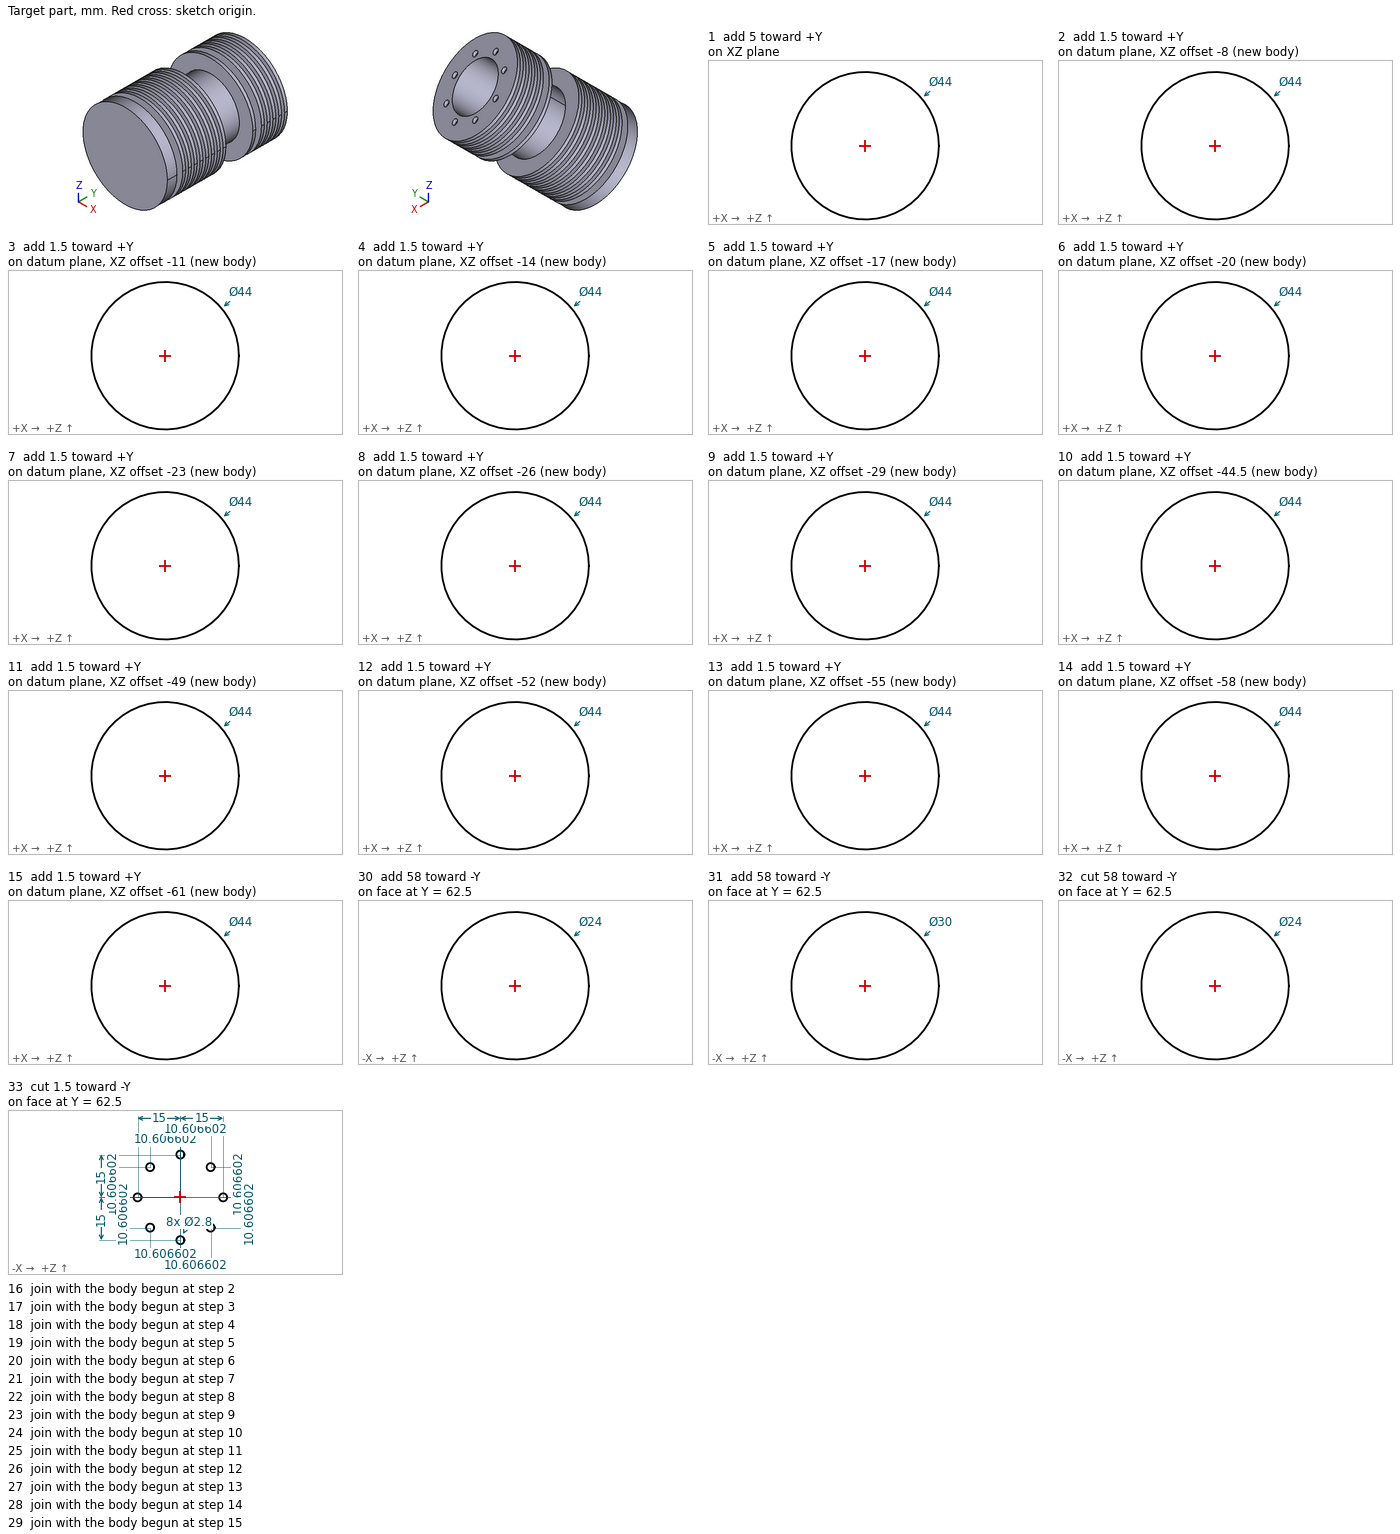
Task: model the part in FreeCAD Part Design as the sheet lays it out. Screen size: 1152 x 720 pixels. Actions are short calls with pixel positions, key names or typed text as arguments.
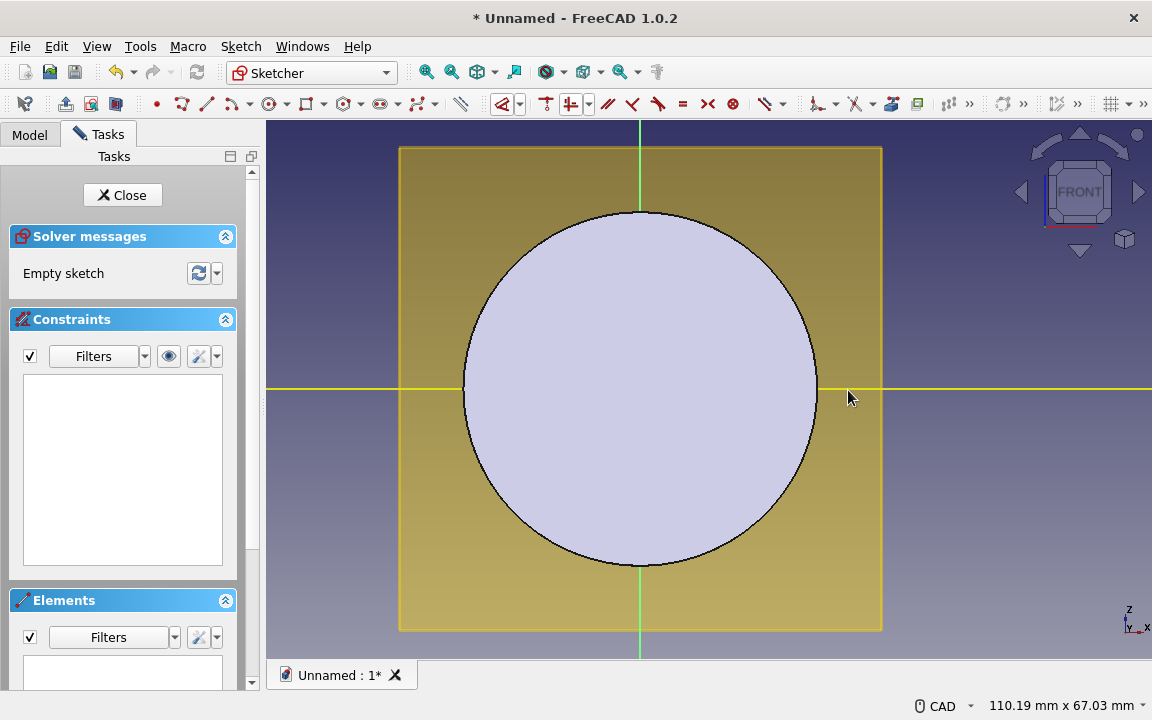
key(g)
key(c)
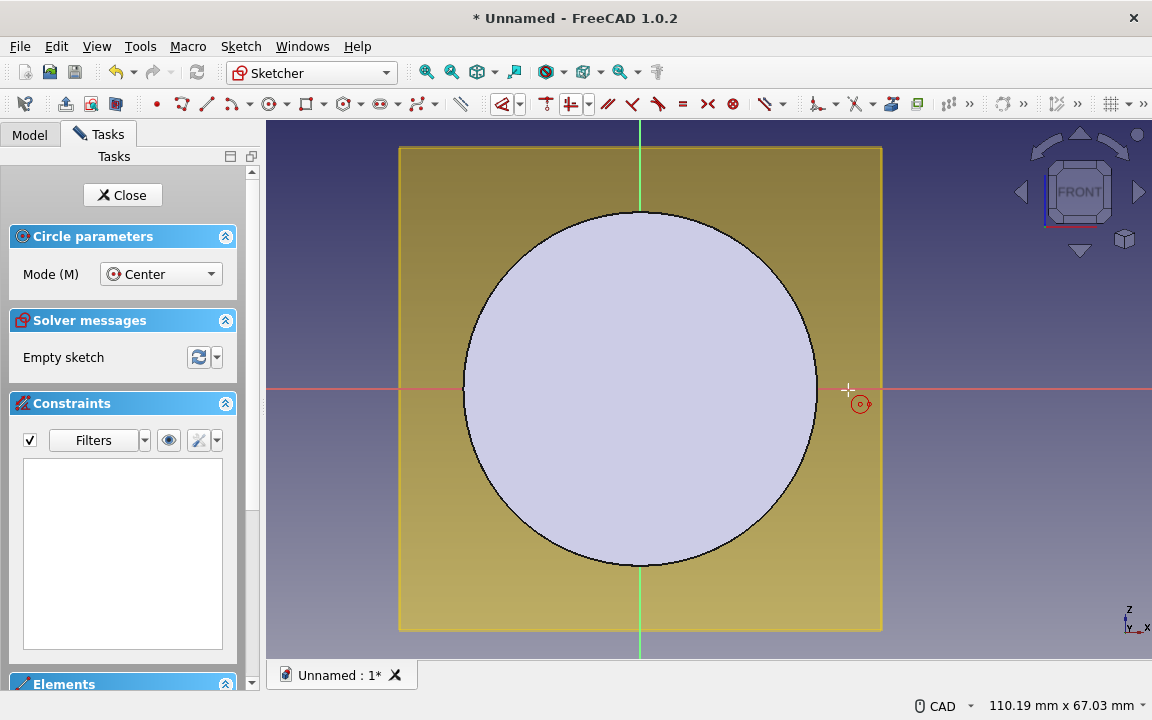
click(640, 389)
click(765, 264)
key(Escape)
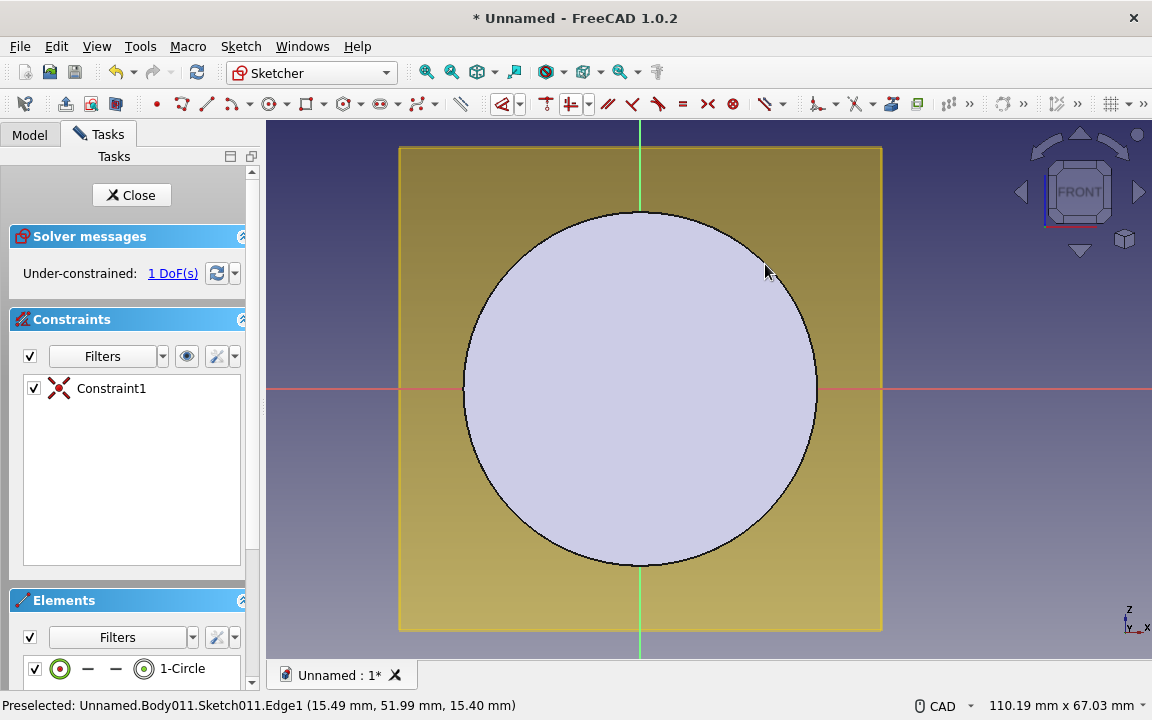
click(764, 264)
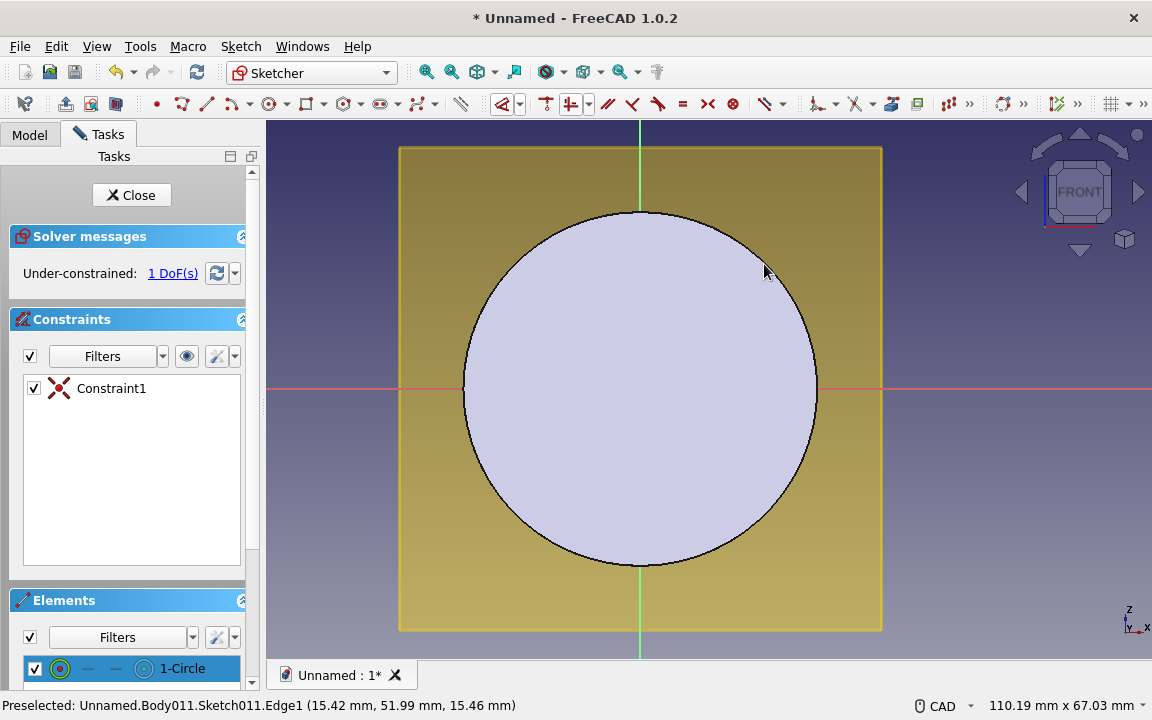
click(520, 104)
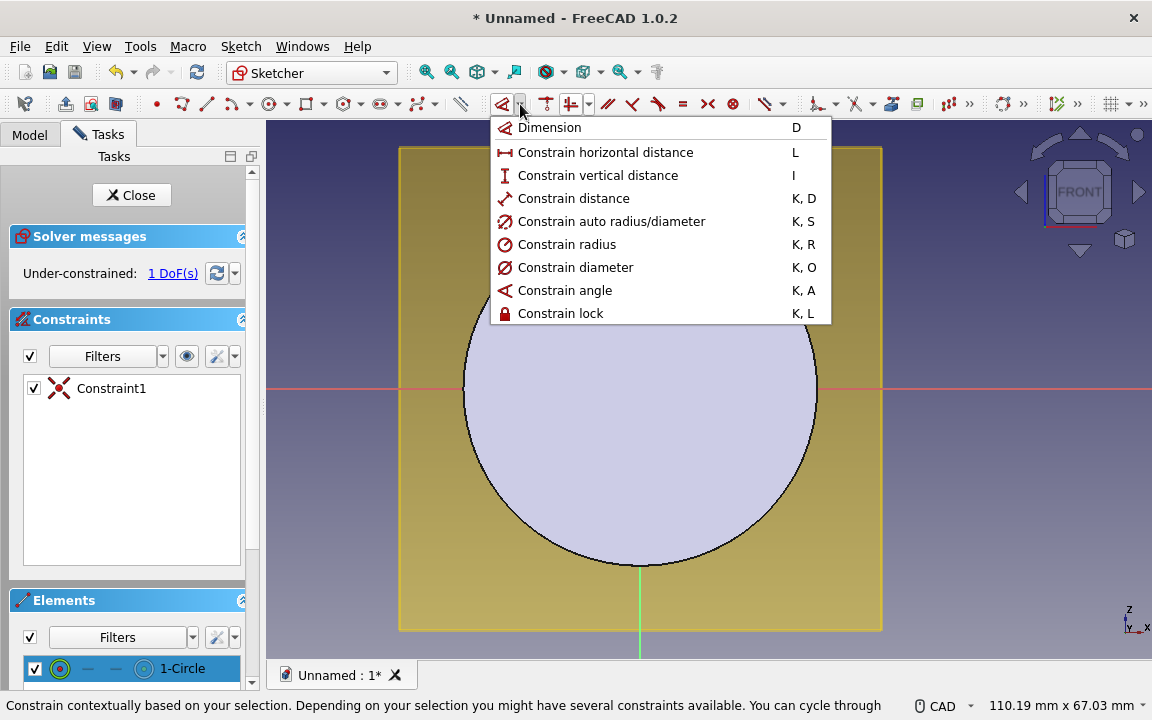
click(661, 268)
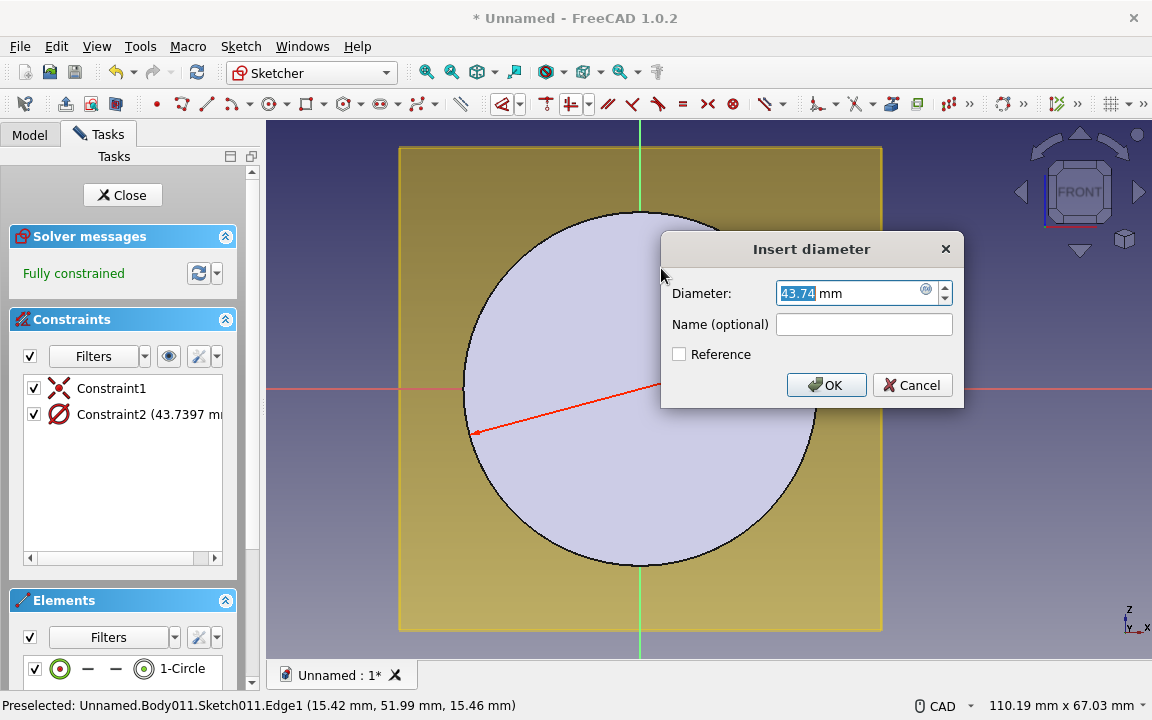
text(44)
key(Return)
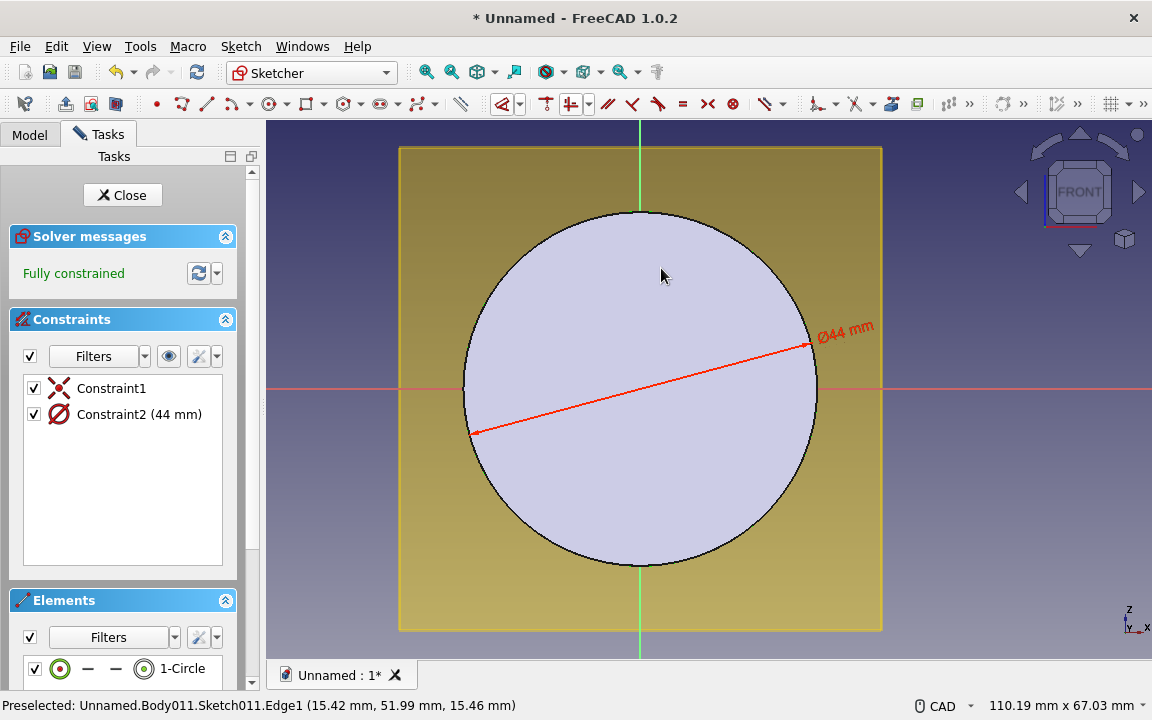
click(123, 195)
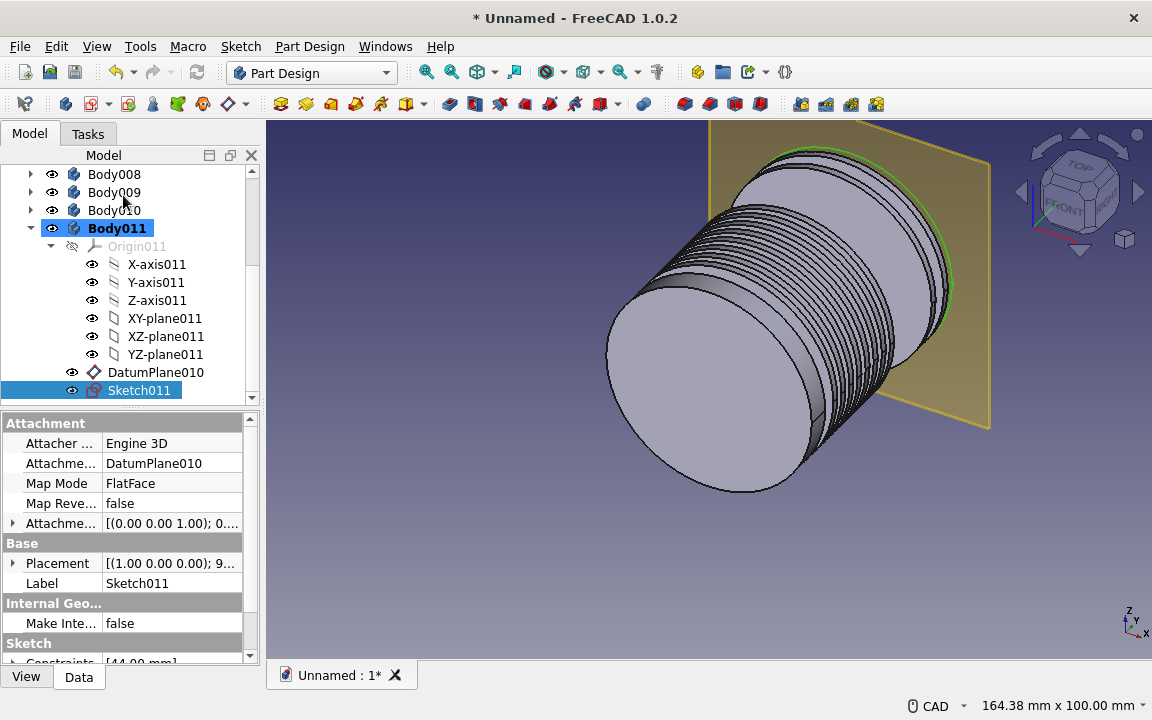
click(281, 104)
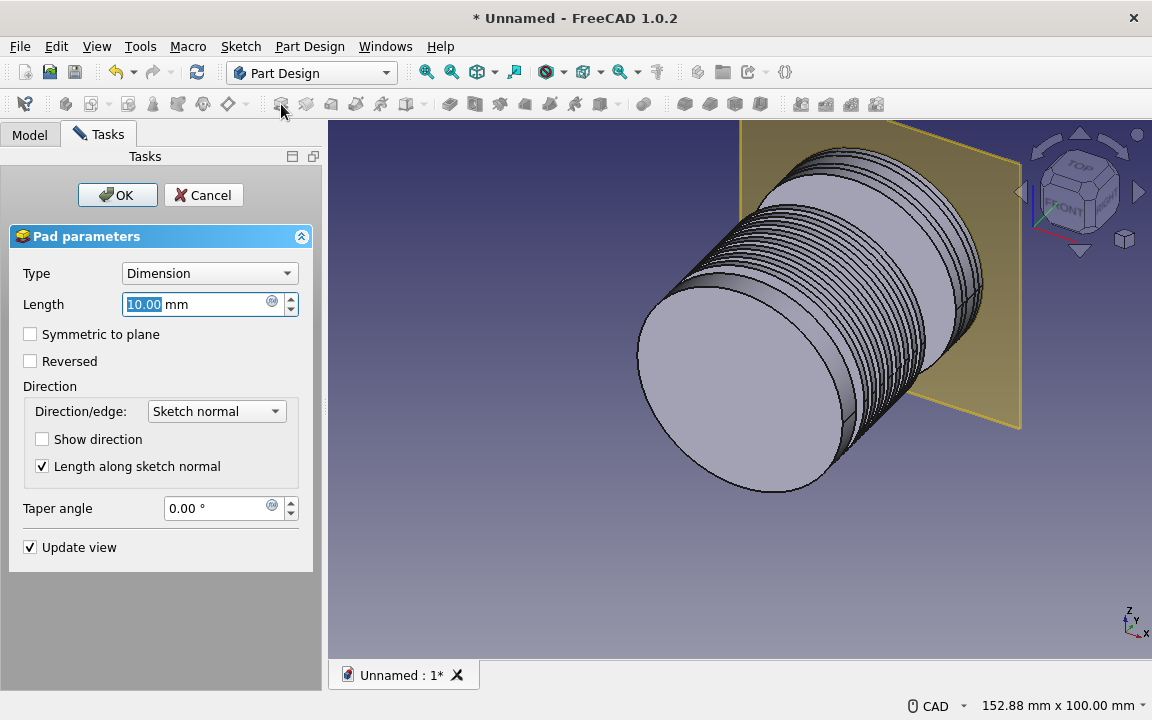
text(1.5)
key(Tab)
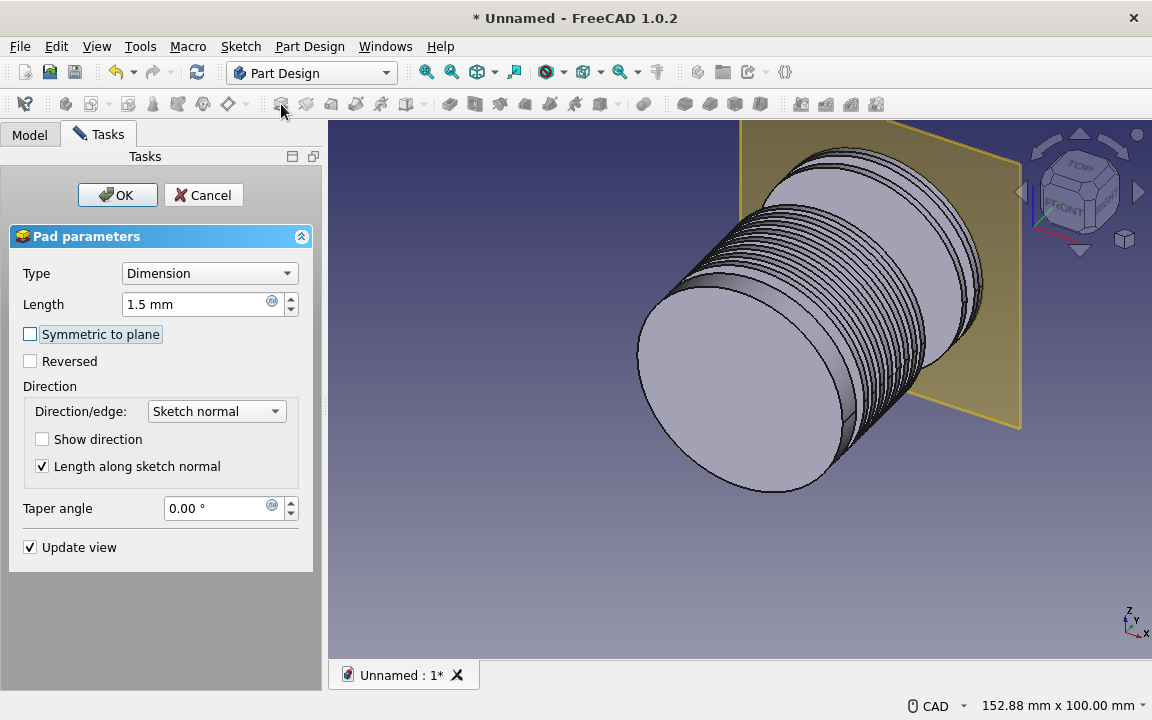
click(31, 361)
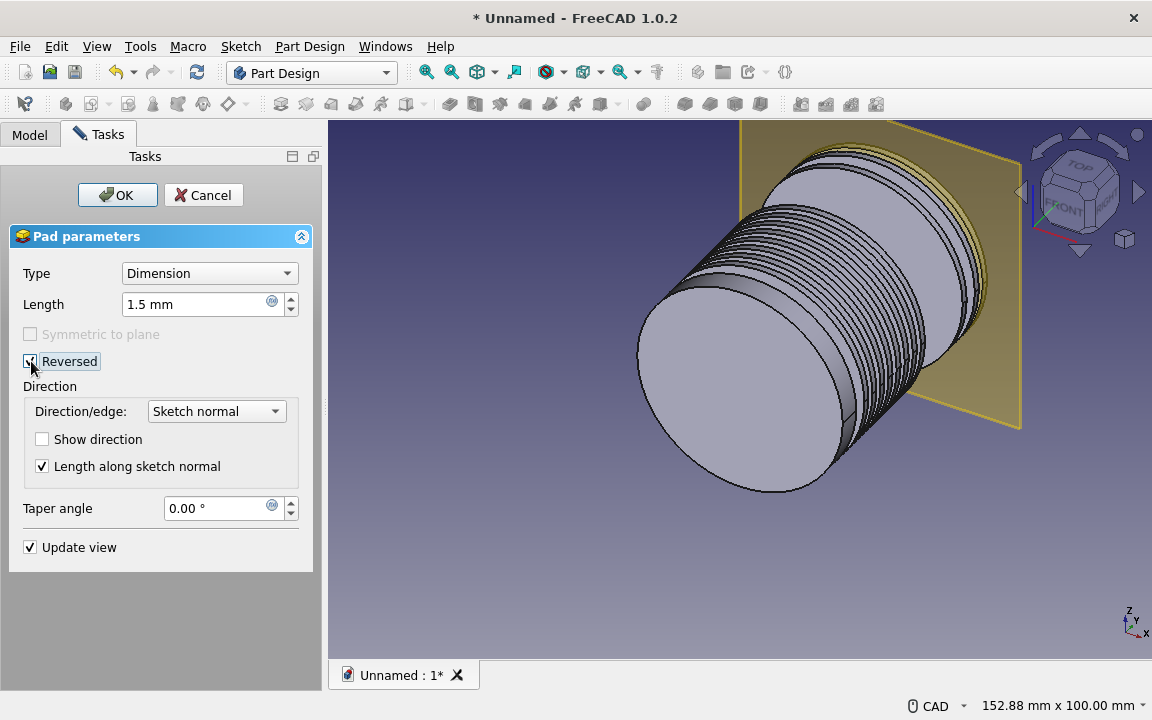
click(118, 195)